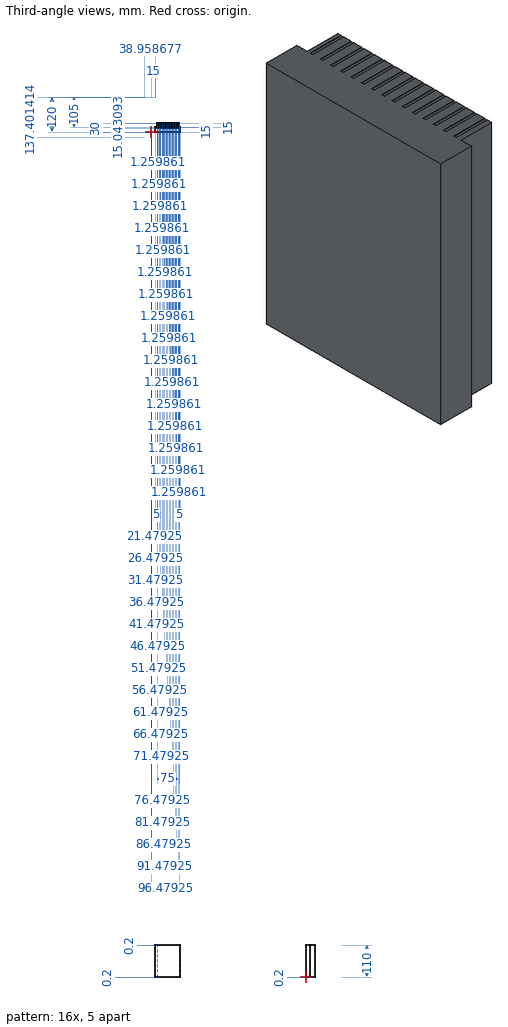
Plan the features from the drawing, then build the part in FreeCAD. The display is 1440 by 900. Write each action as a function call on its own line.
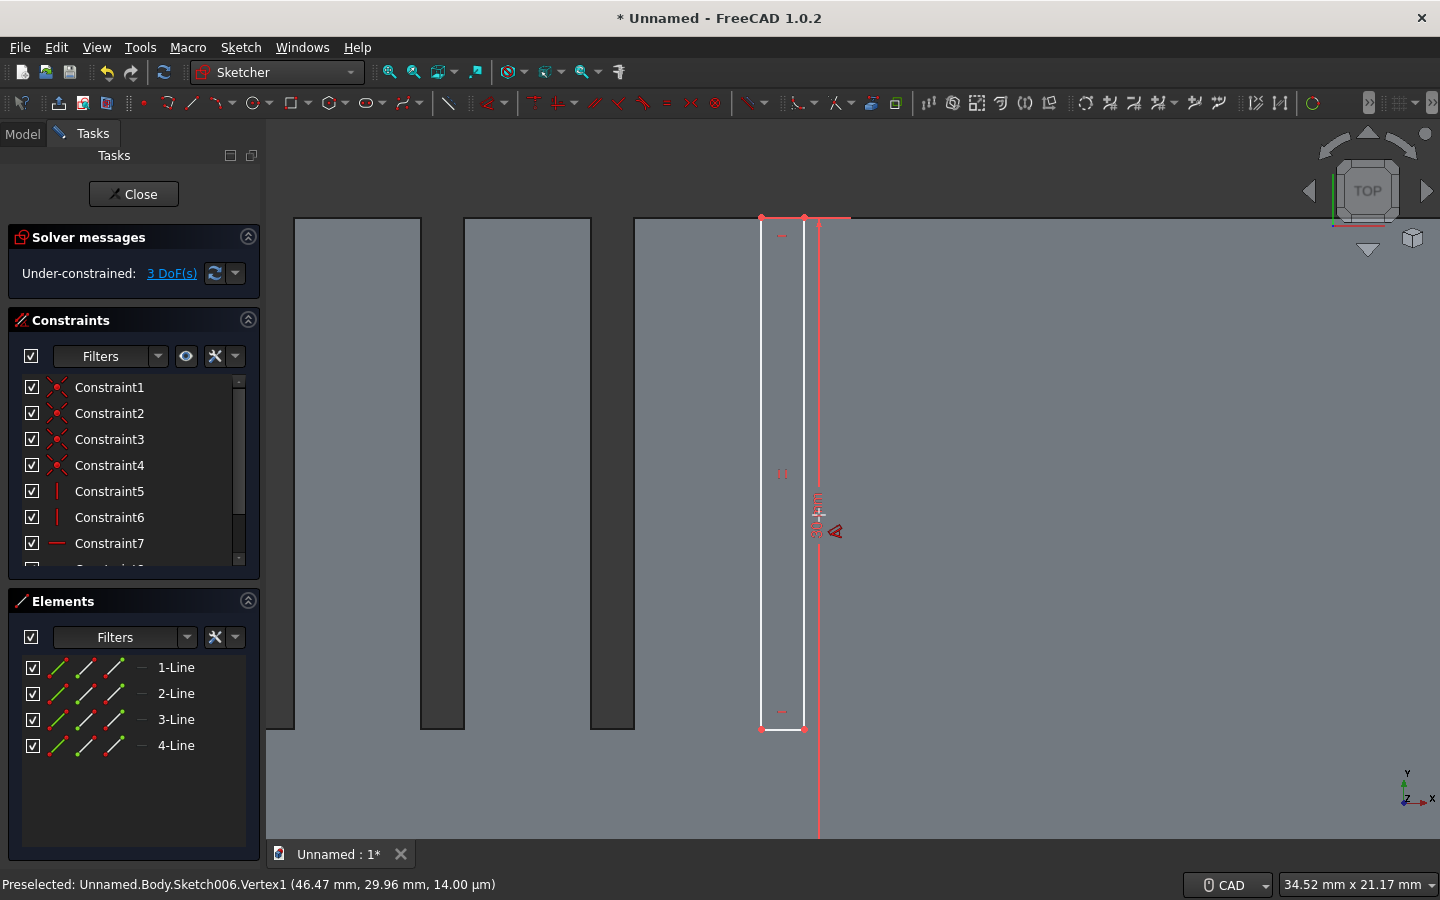
click(774, 730)
click(782, 764)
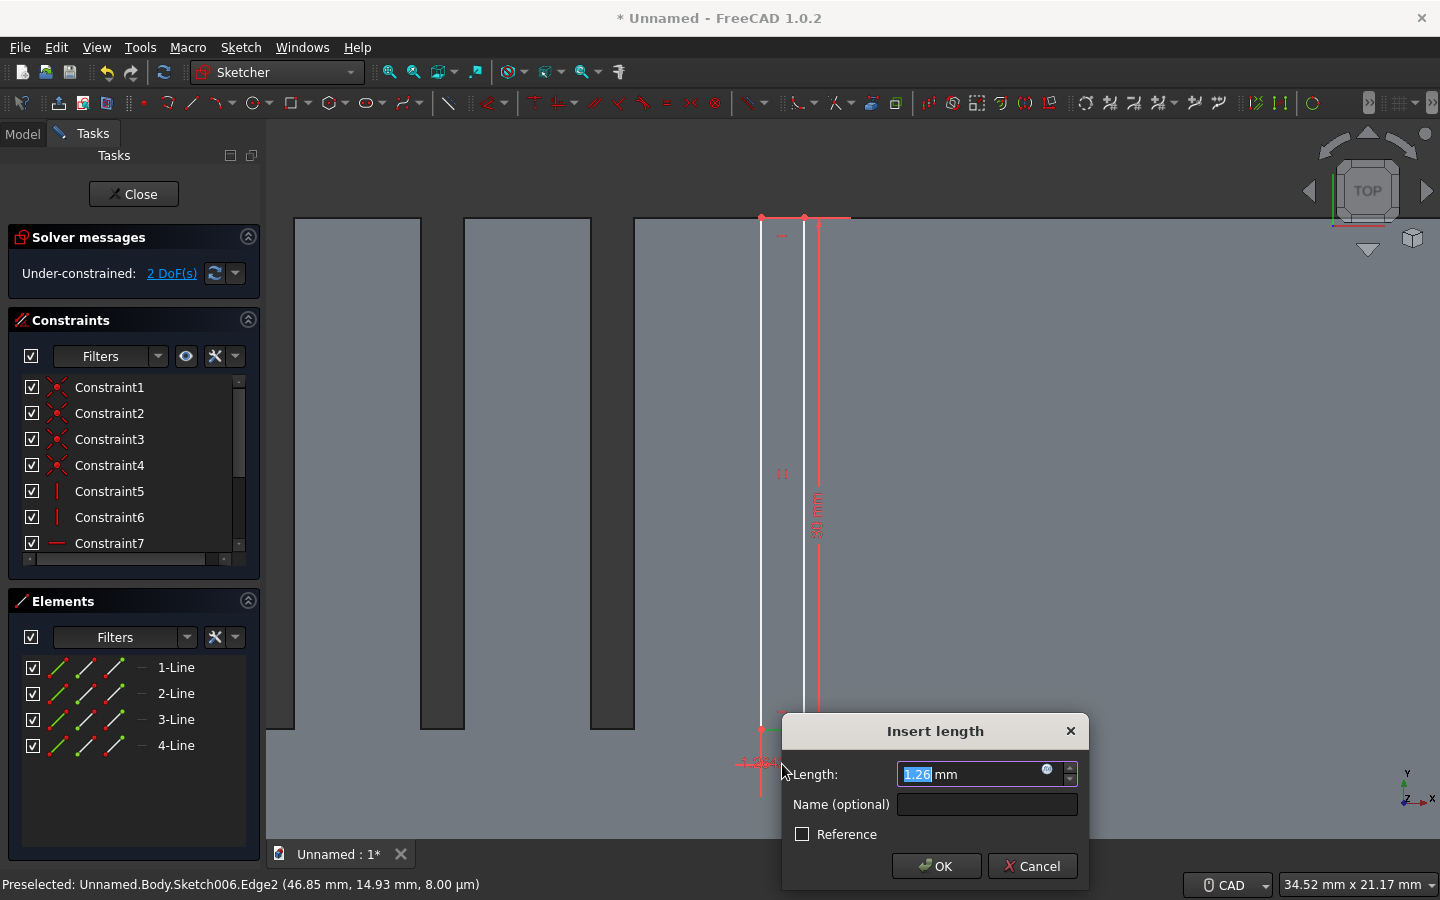
text(1.259861)
key(Return)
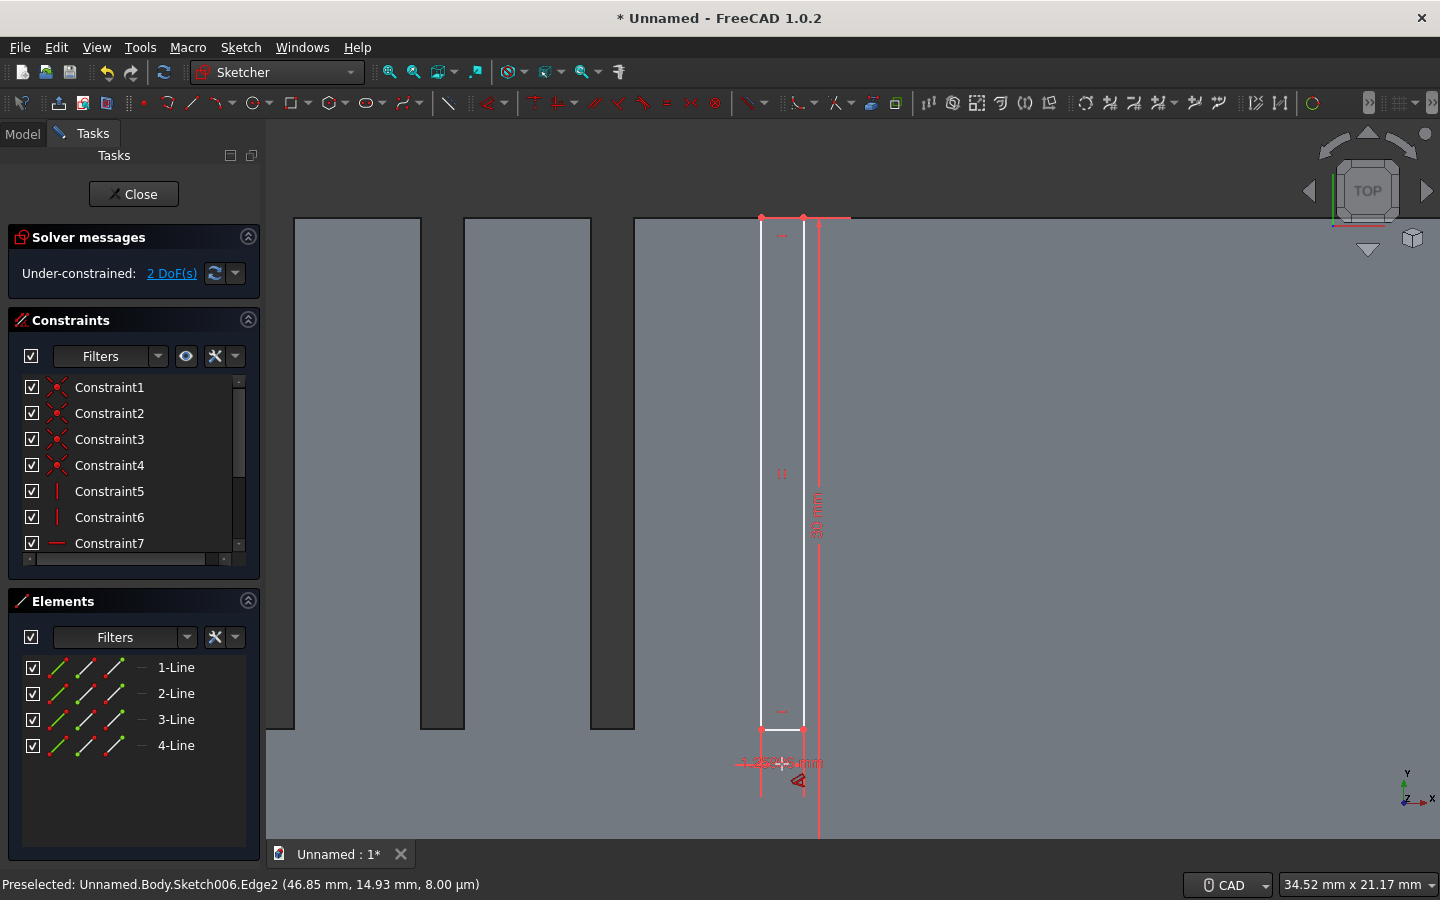
click(761, 371)
click(727, 474)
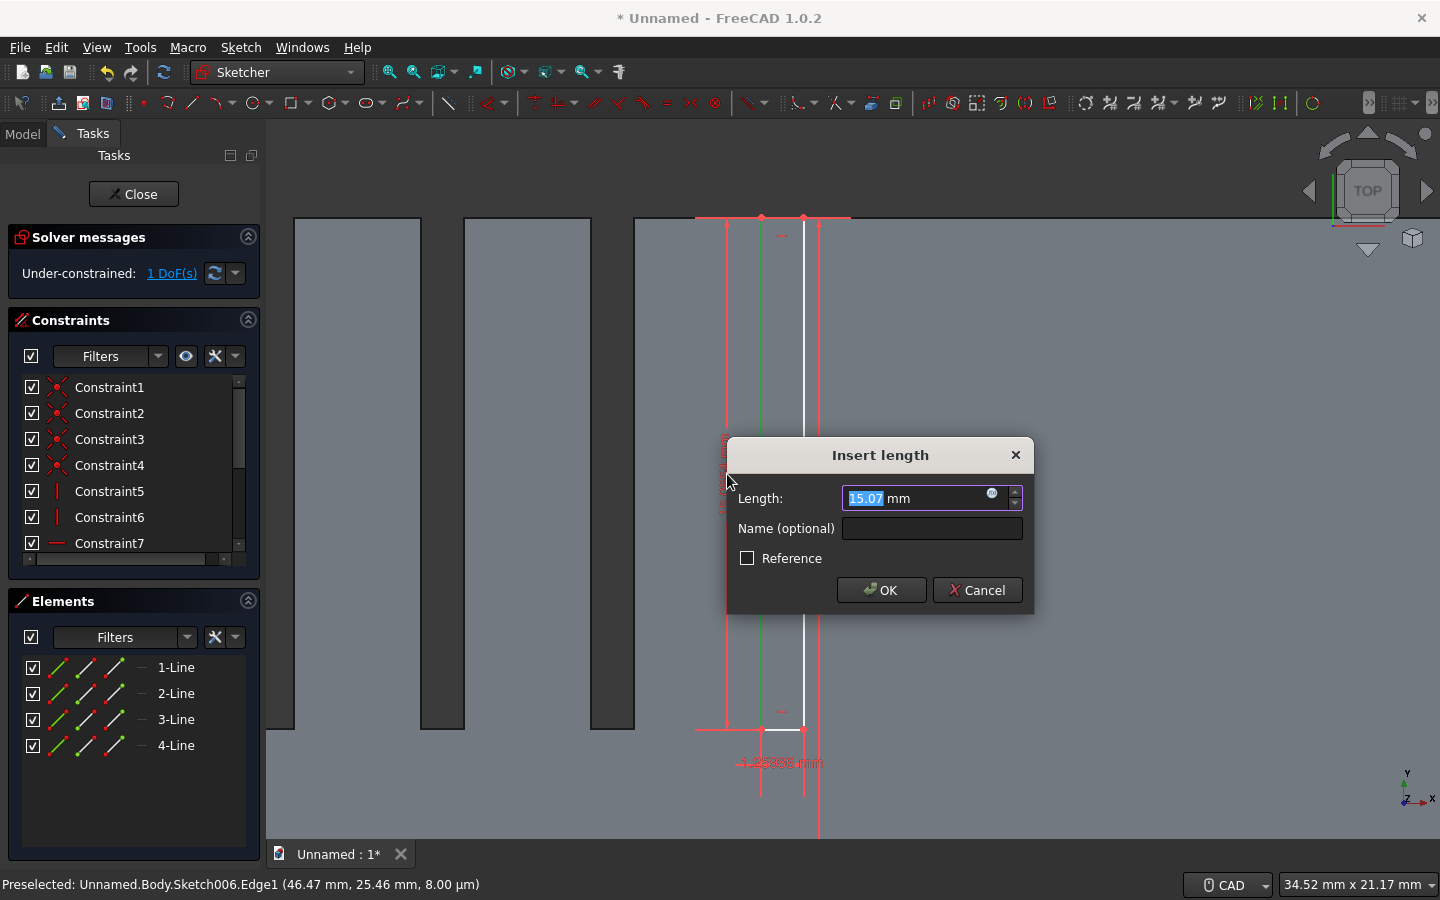
text(15.043093)
key(Return)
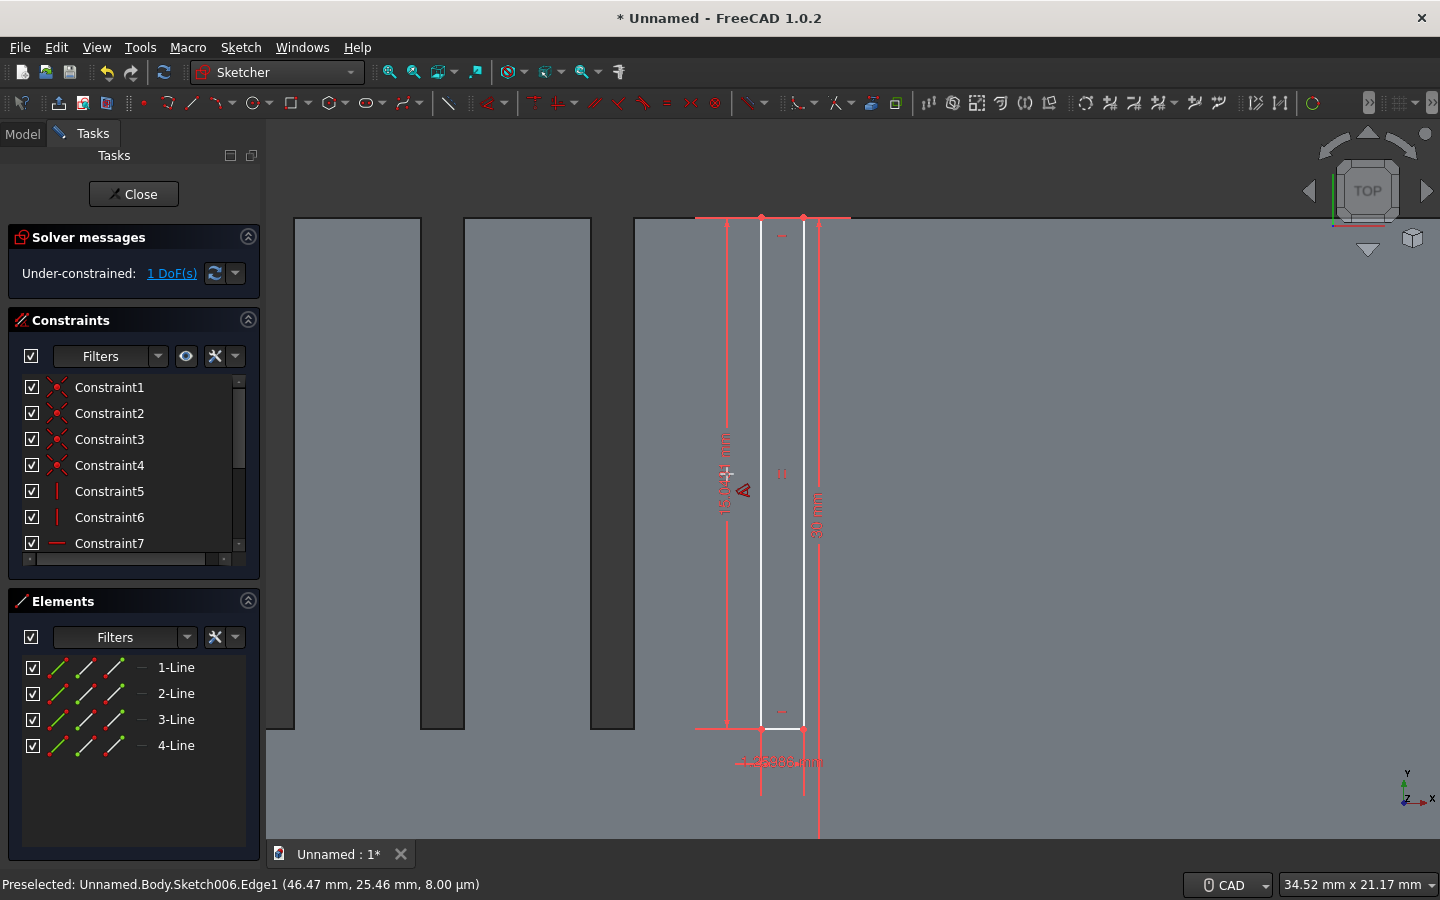
click(761, 218)
click(527, 184)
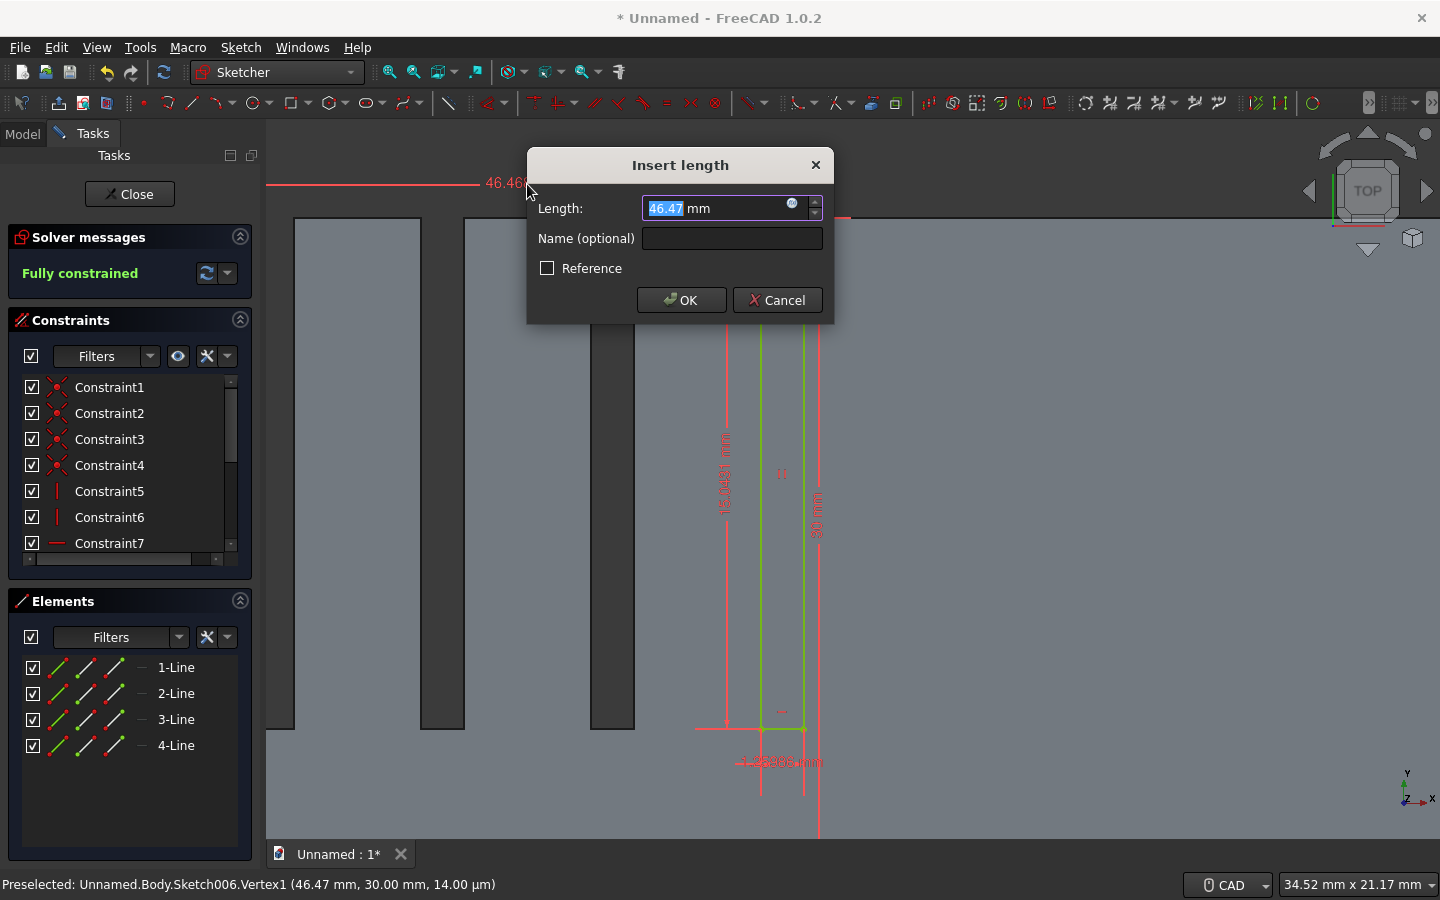
text(46.47925)
key(Return)
key(Escape)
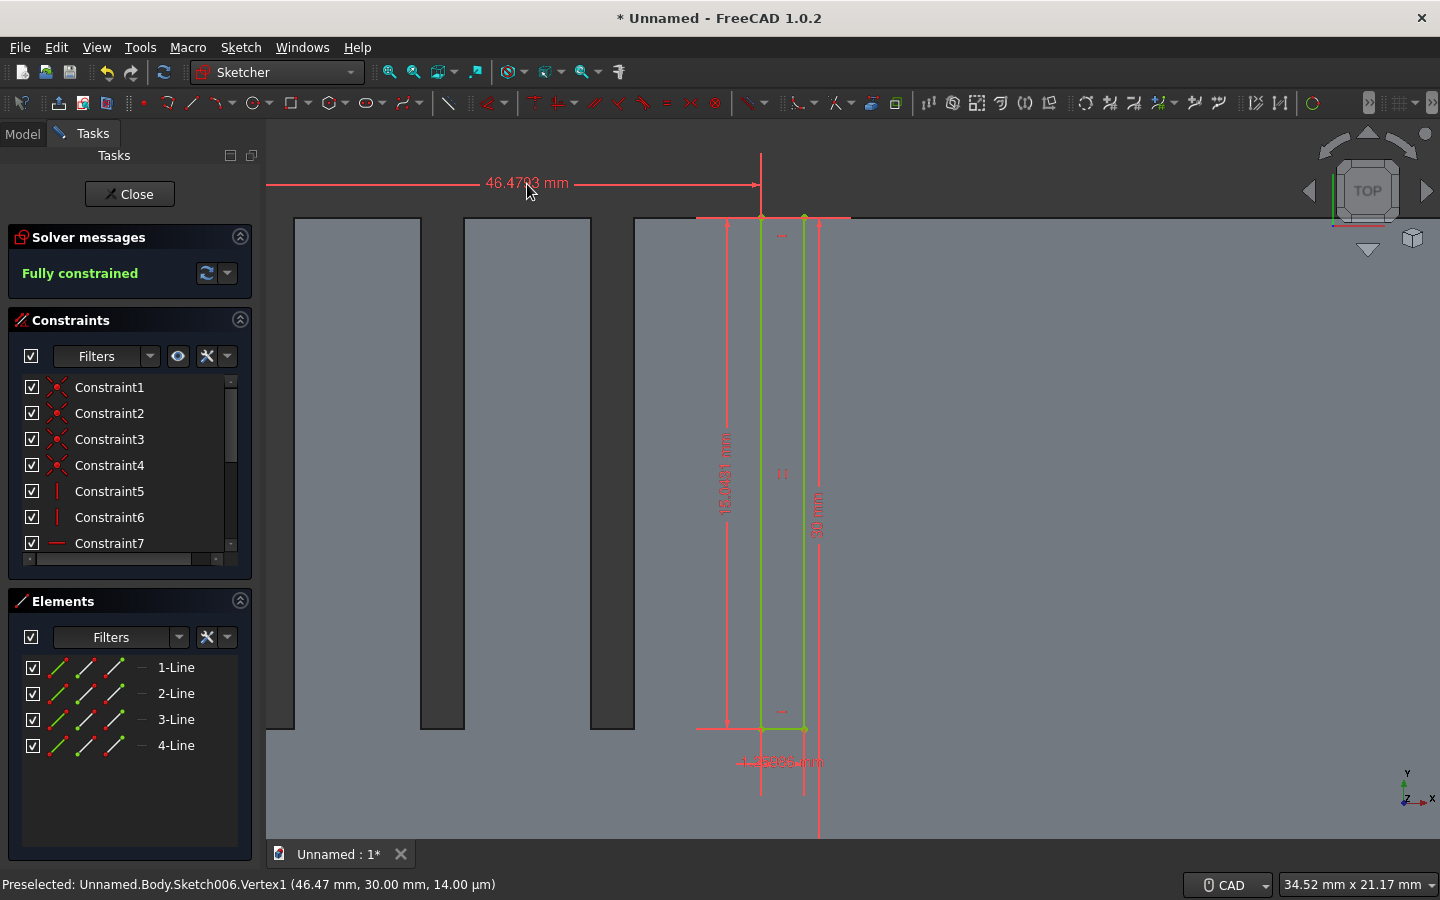
click(130, 194)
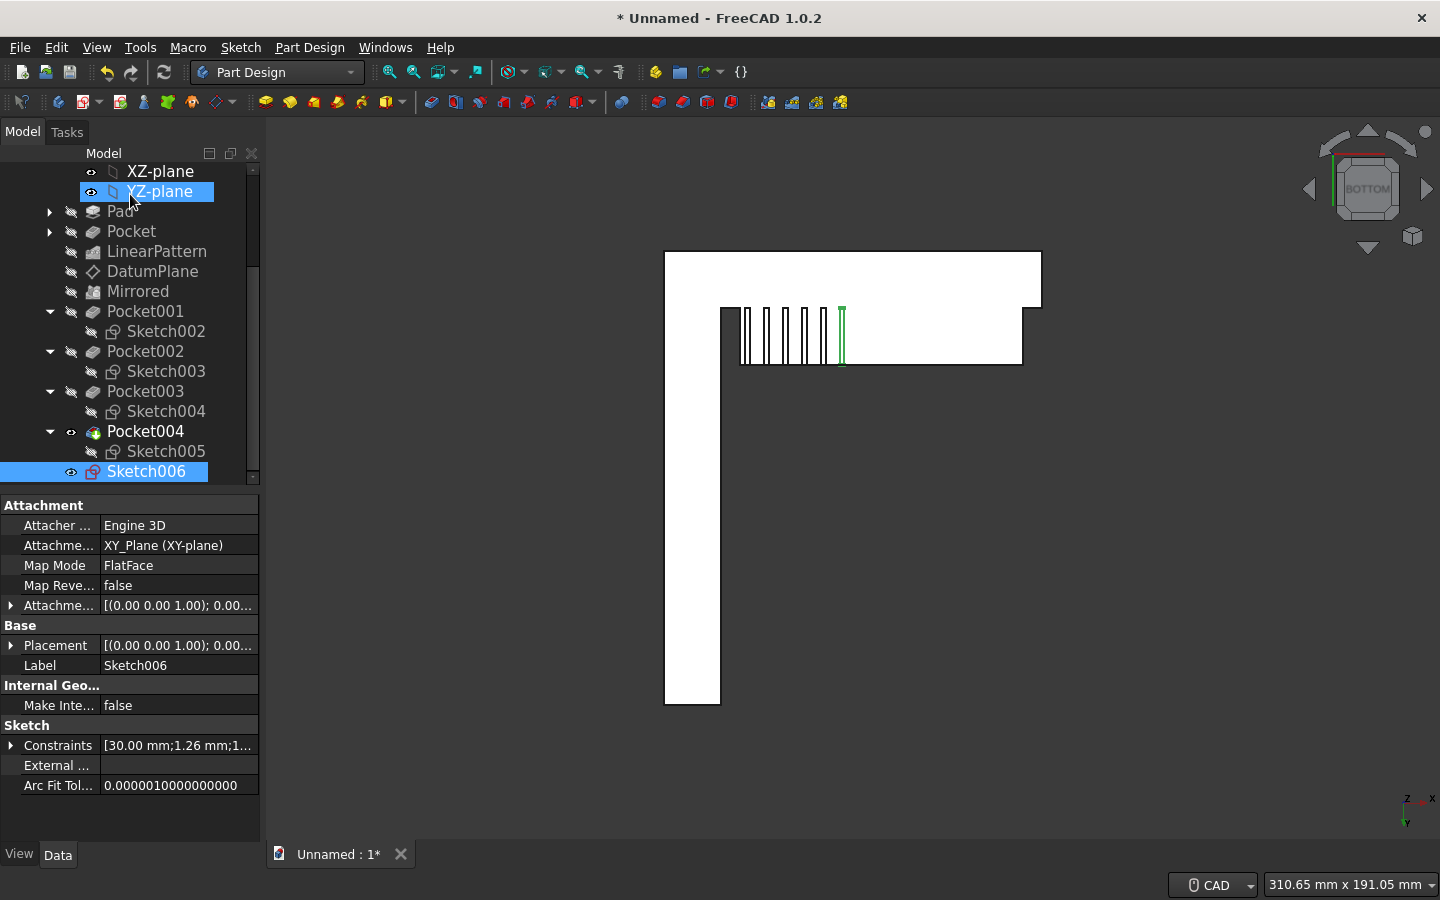
click(432, 102)